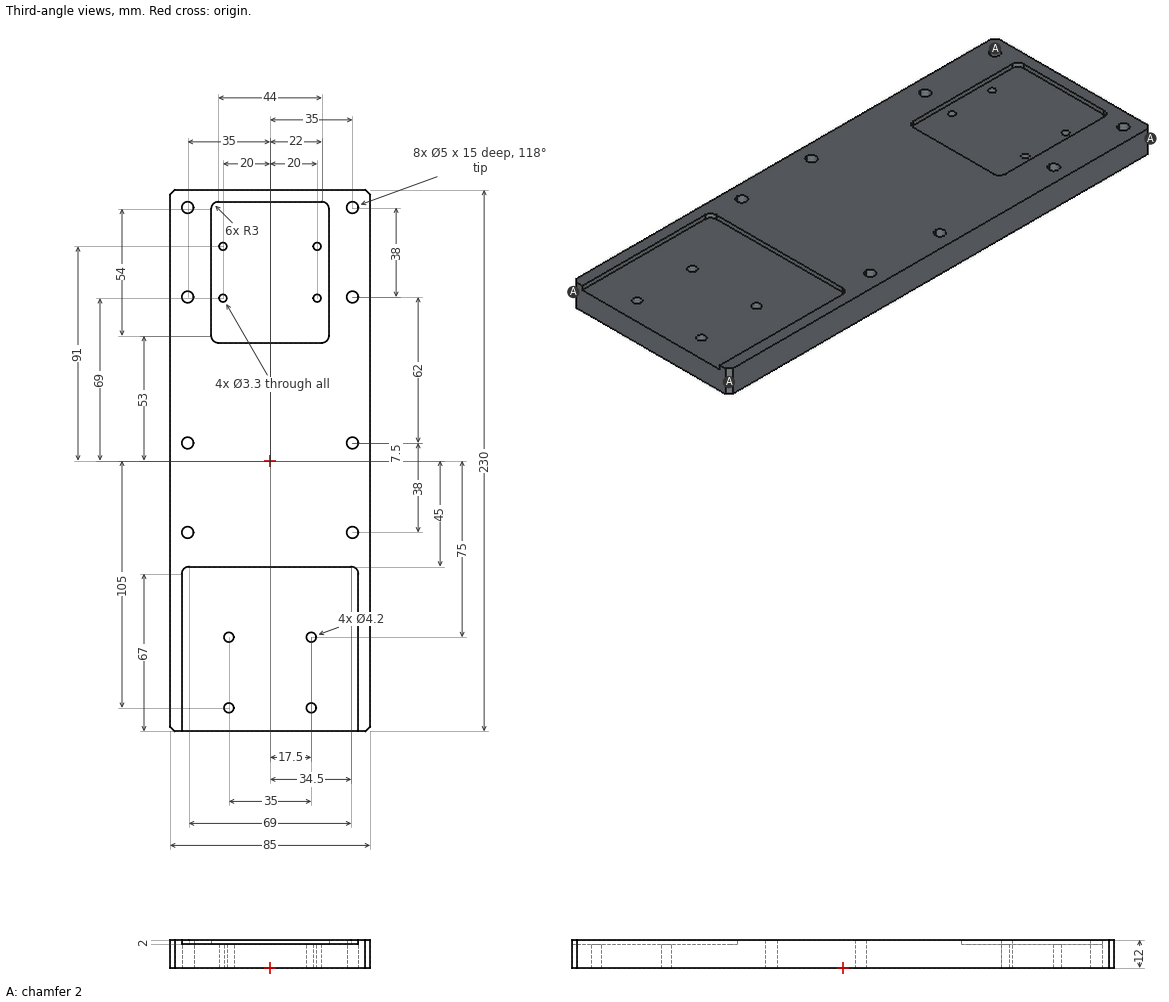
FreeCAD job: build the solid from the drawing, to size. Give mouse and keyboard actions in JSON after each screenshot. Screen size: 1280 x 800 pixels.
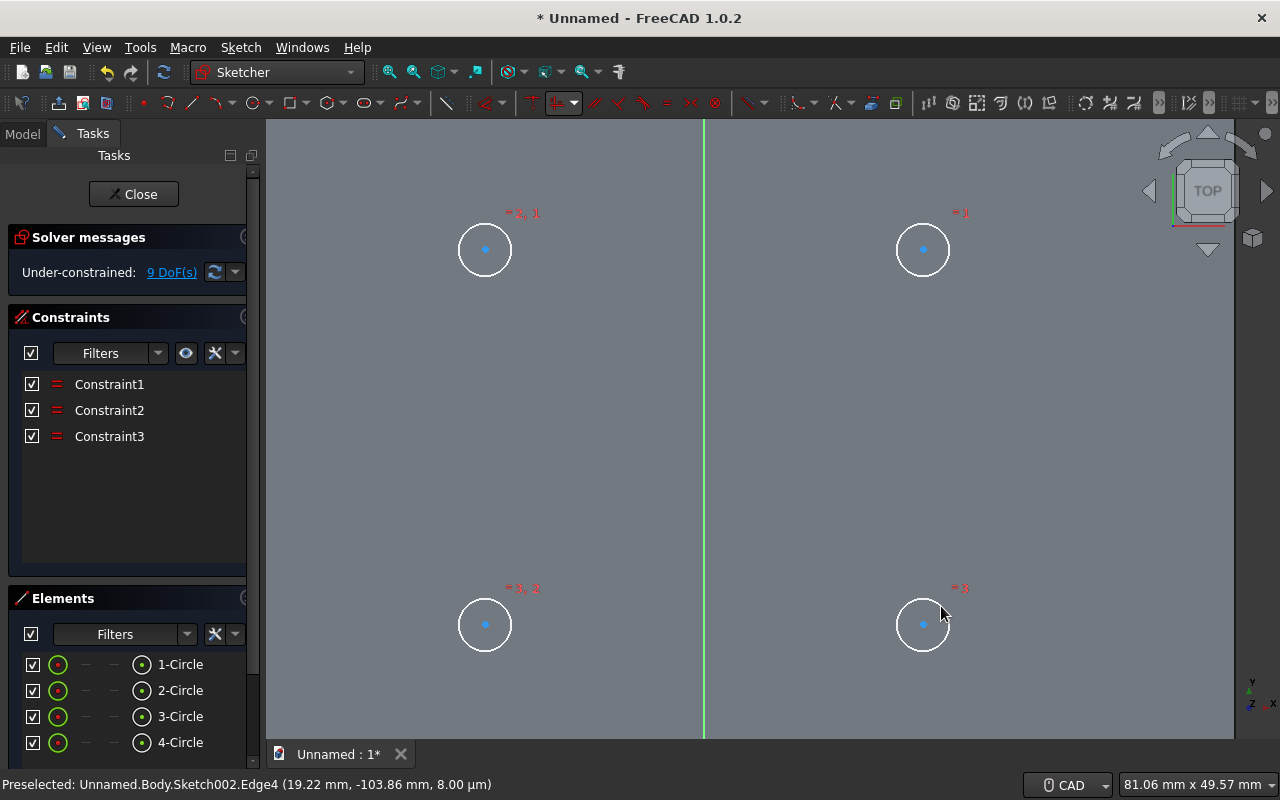
{"action": "left_click", "coordinate": [923, 250]}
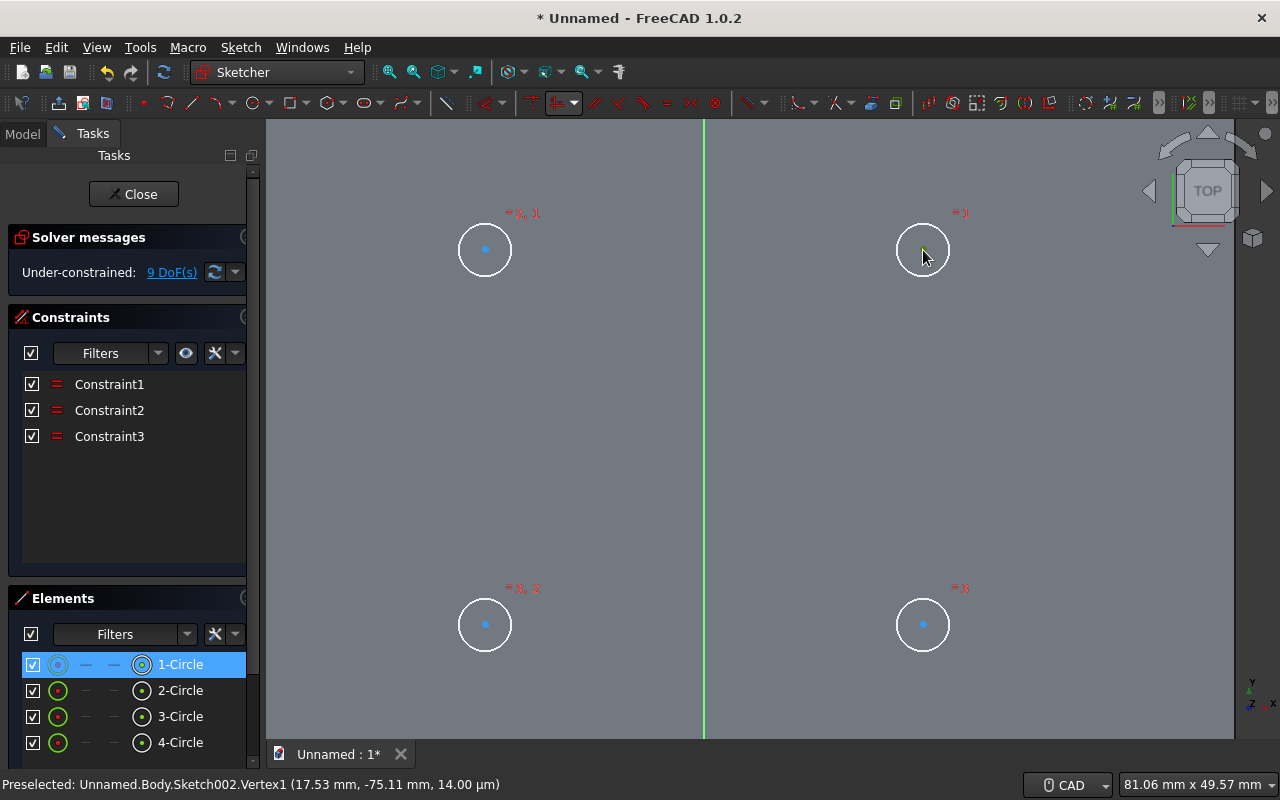
{"action": "left_click", "coordinate": [485, 250]}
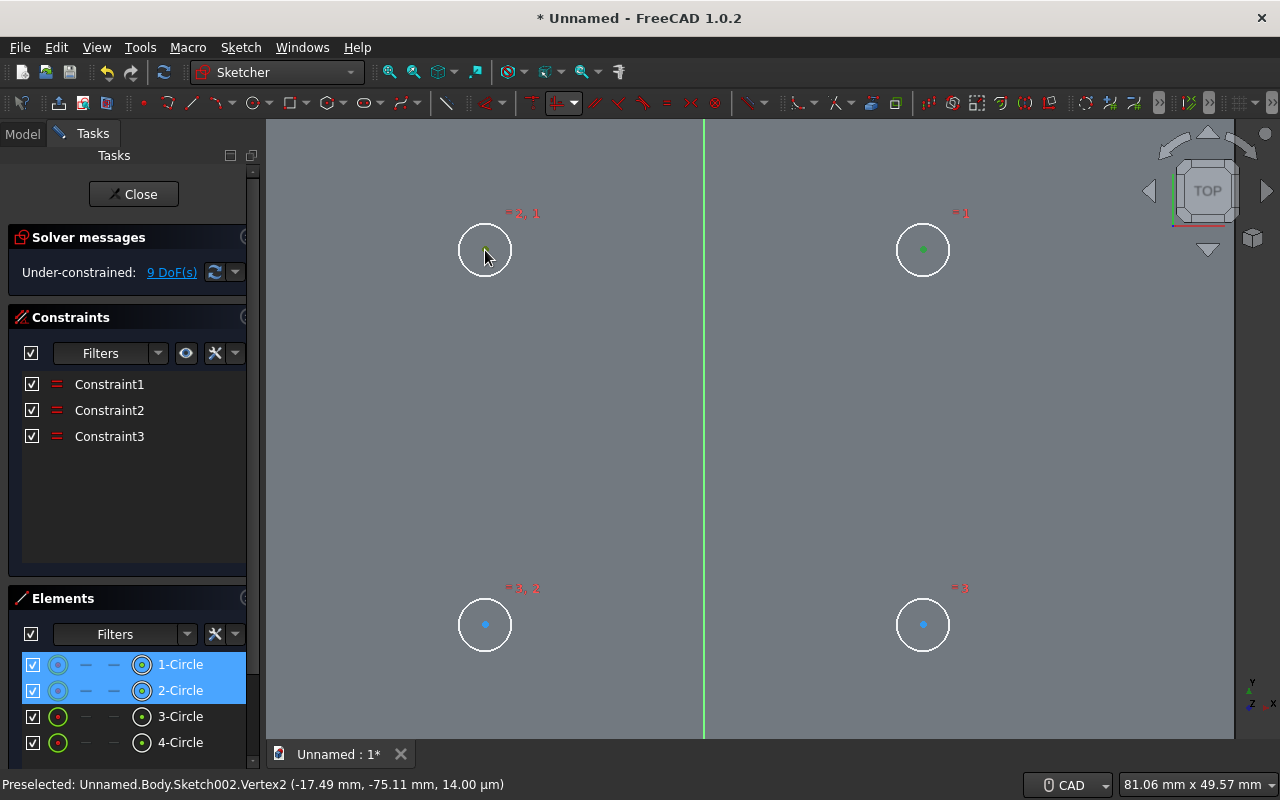
{"action": "key", "text": "h"}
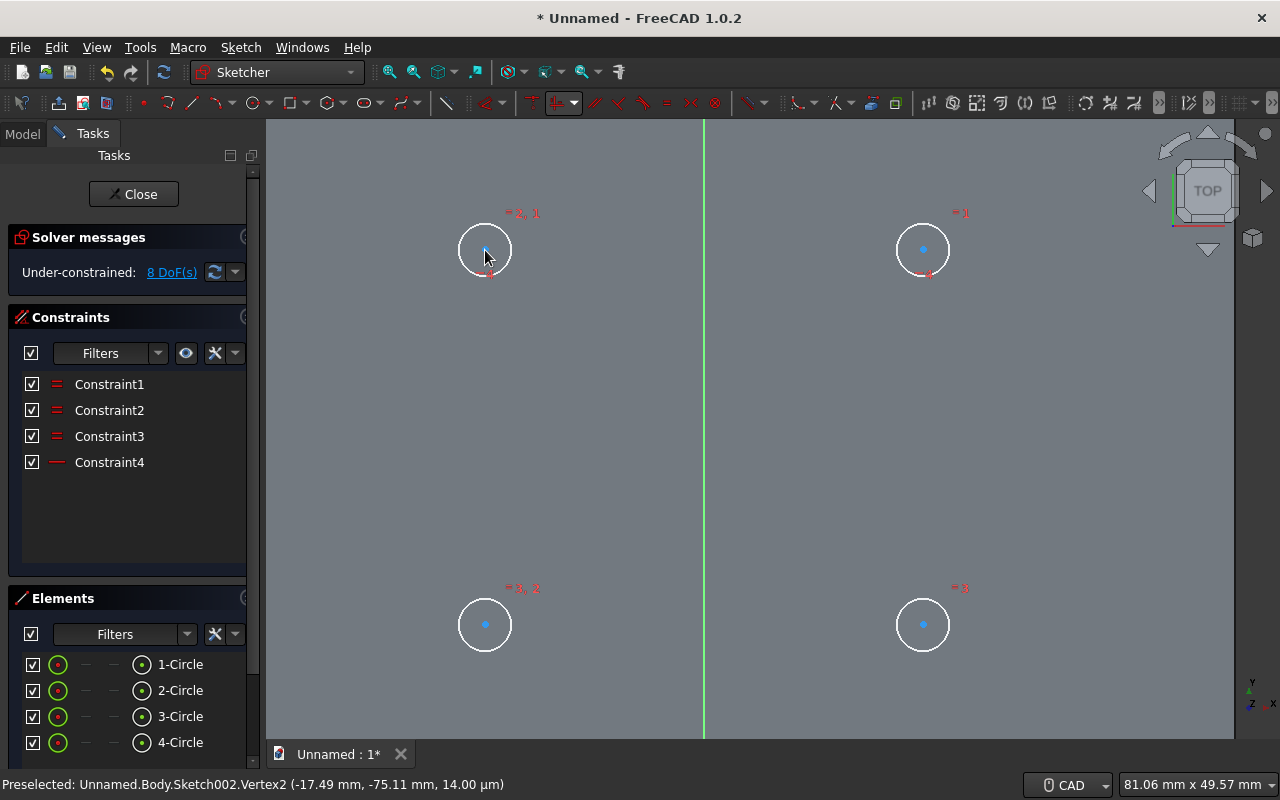
{"action": "left_click", "coordinate": [485, 250]}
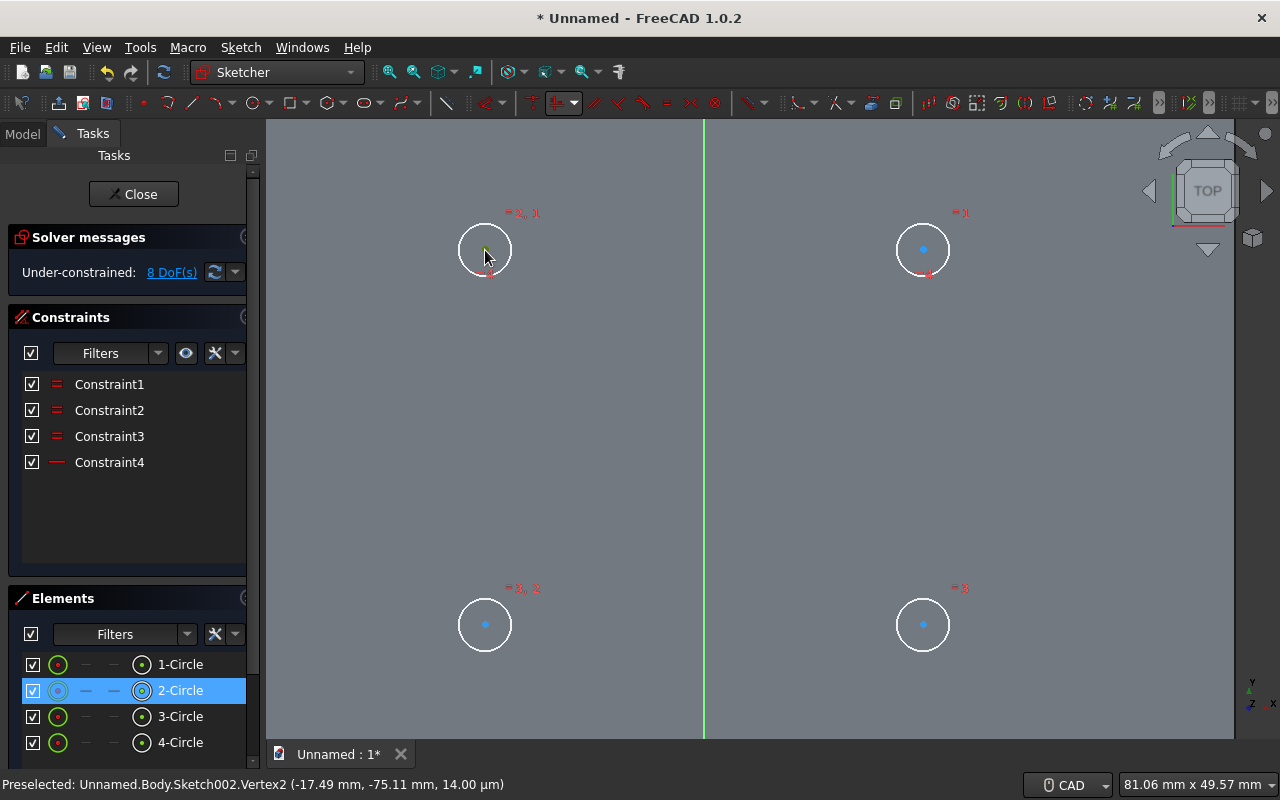
{"action": "left_click", "coordinate": [485, 625]}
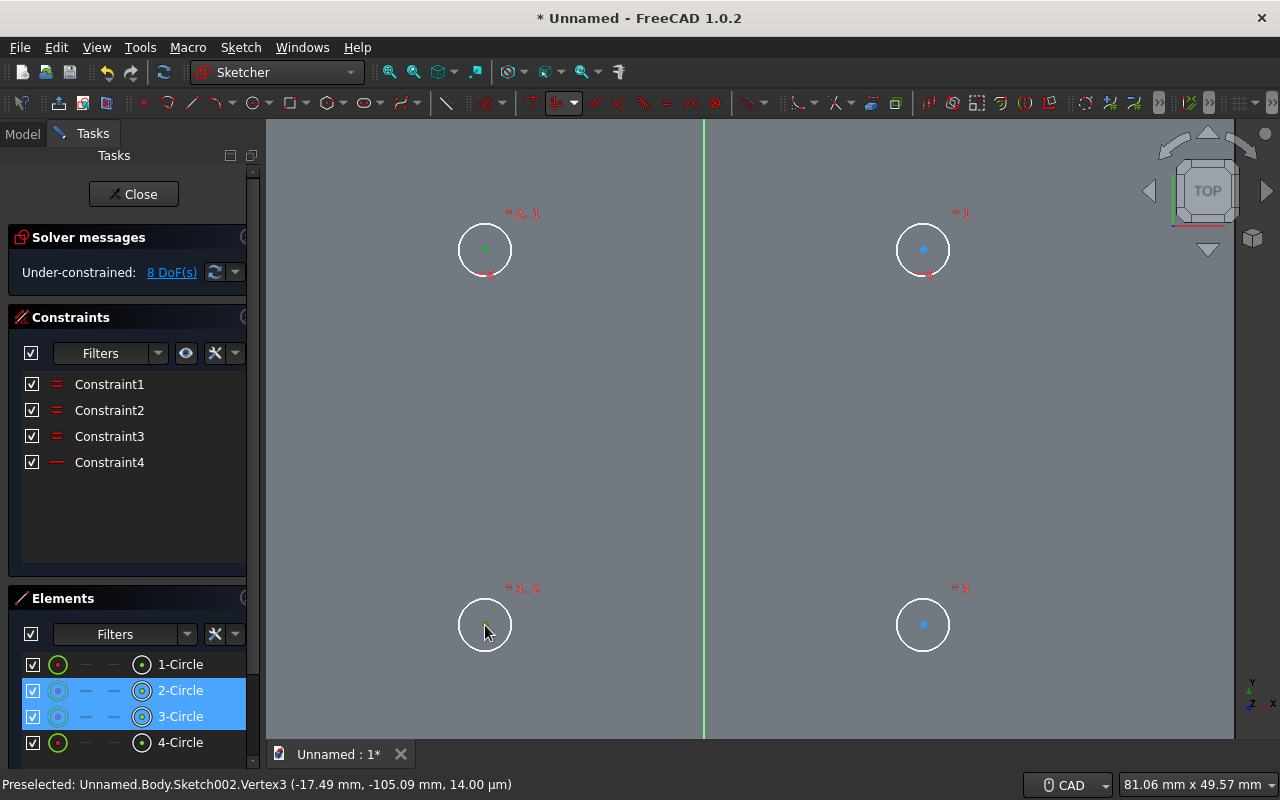
{"action": "key", "text": "v"}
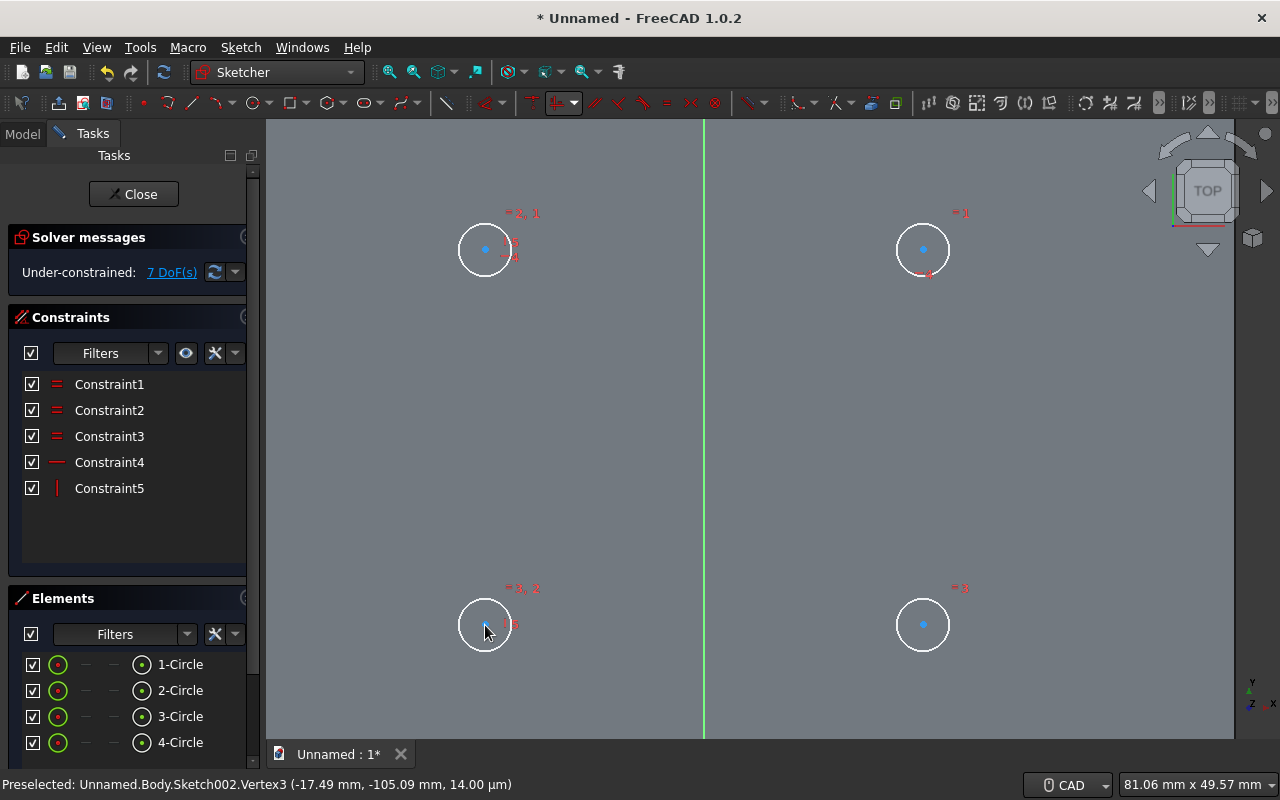
{"action": "left_click", "coordinate": [923, 250]}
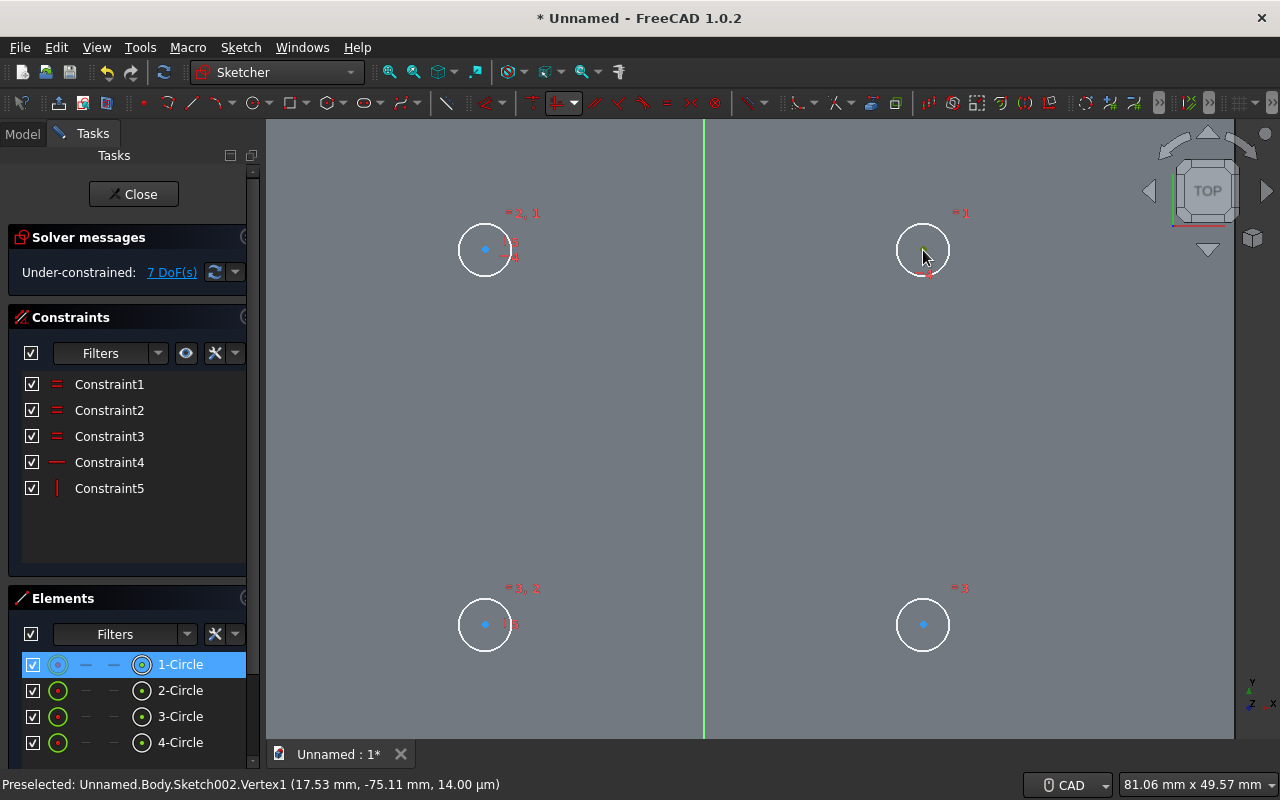
{"action": "left_click", "coordinate": [923, 625]}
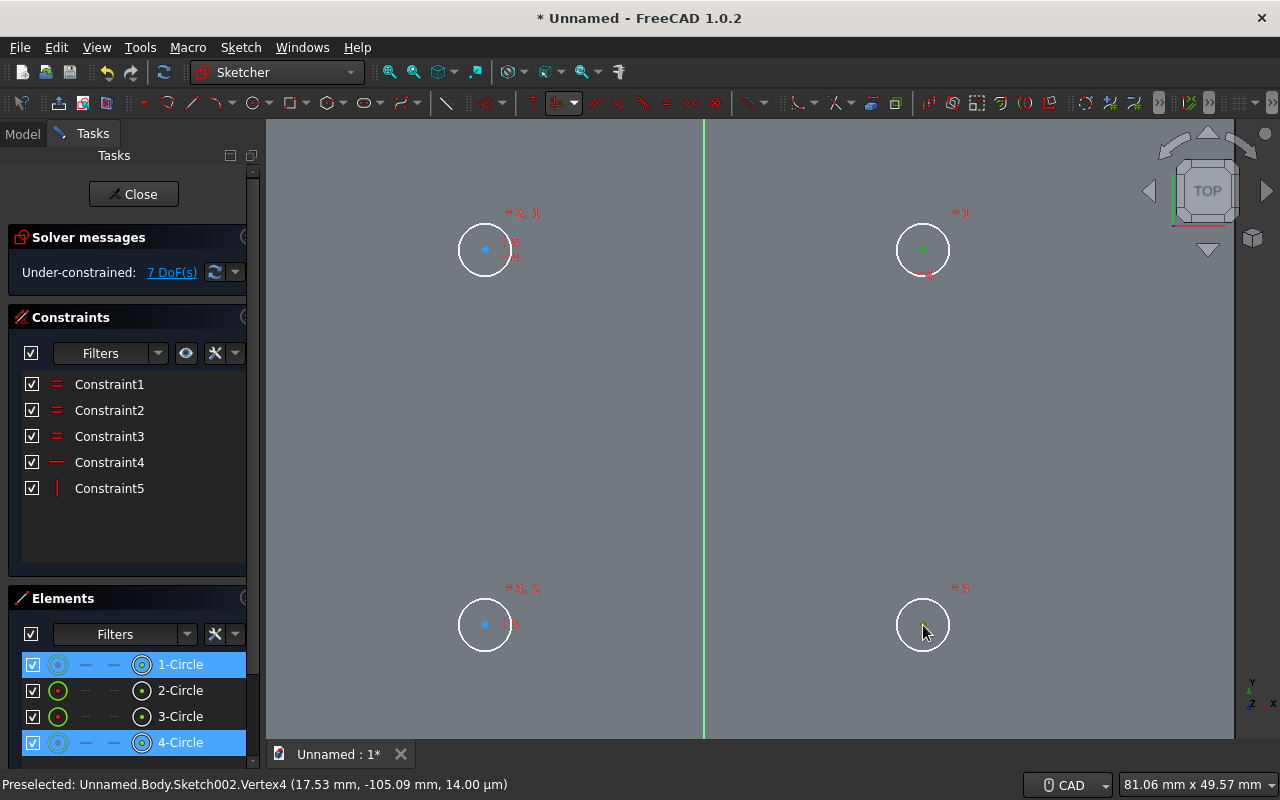
{"action": "key", "text": "v"}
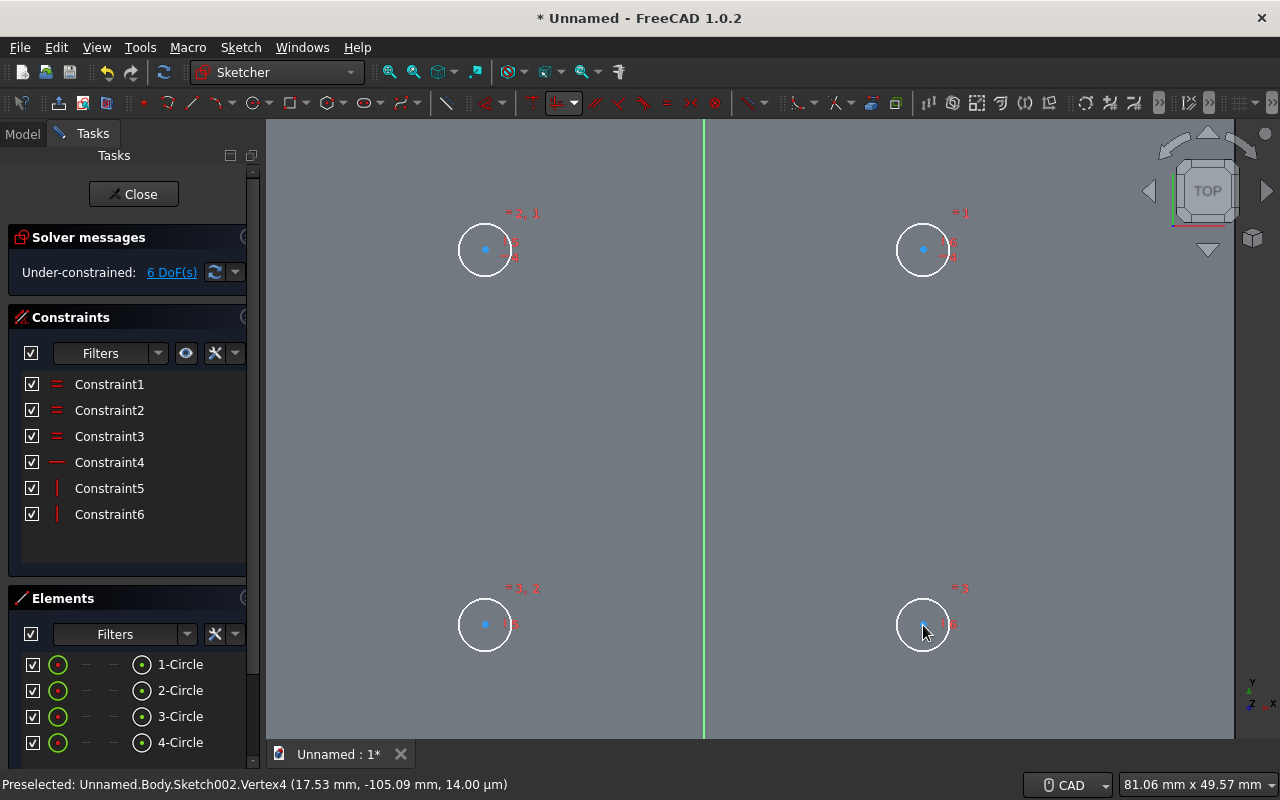
{"action": "left_click", "coordinate": [485, 625]}